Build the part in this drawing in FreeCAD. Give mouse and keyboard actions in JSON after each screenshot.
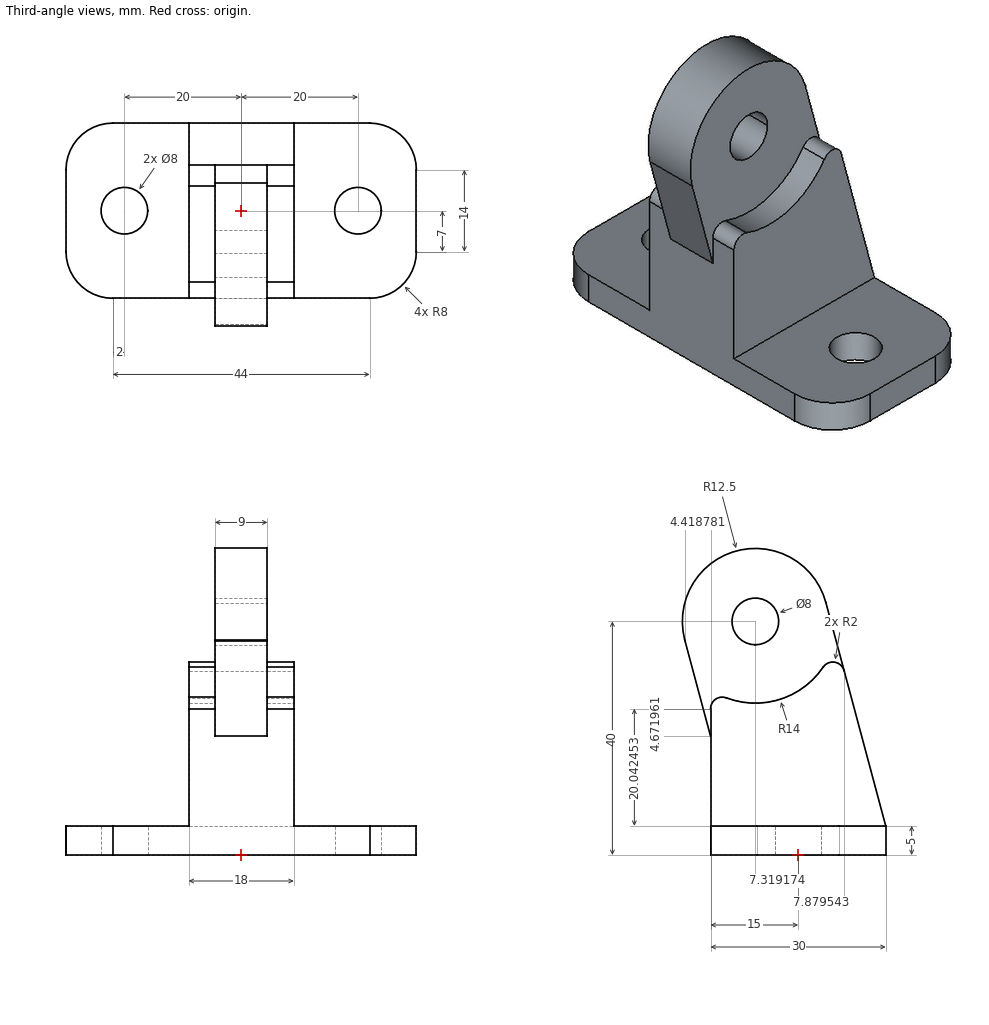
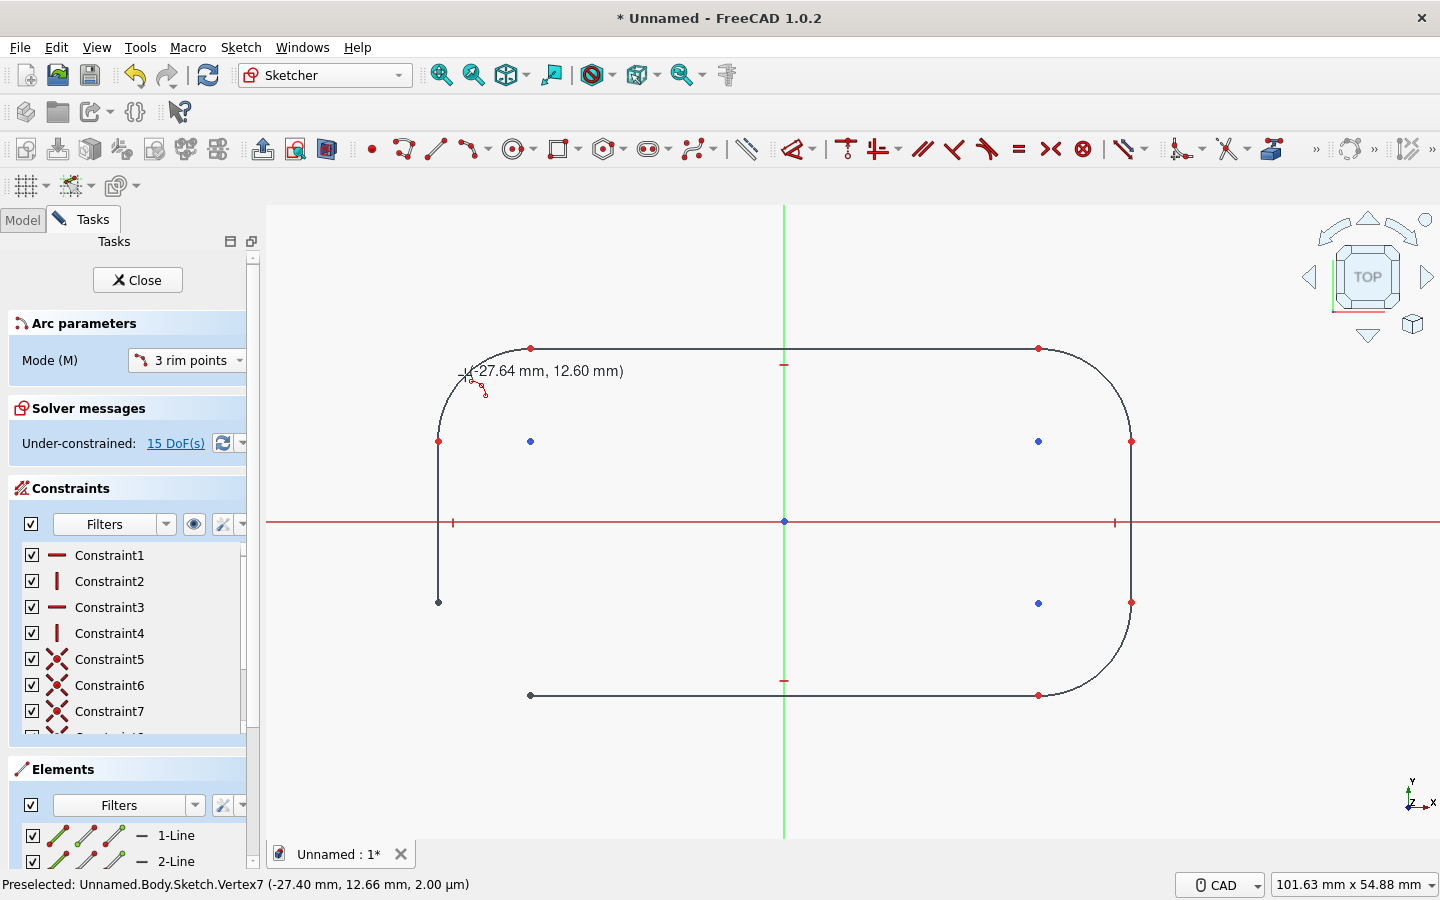
{"action": "left_click", "coordinate": [438, 603]}
{"action": "left_click", "coordinate": [530, 696]}
{"action": "left_click", "coordinate": [465, 668]}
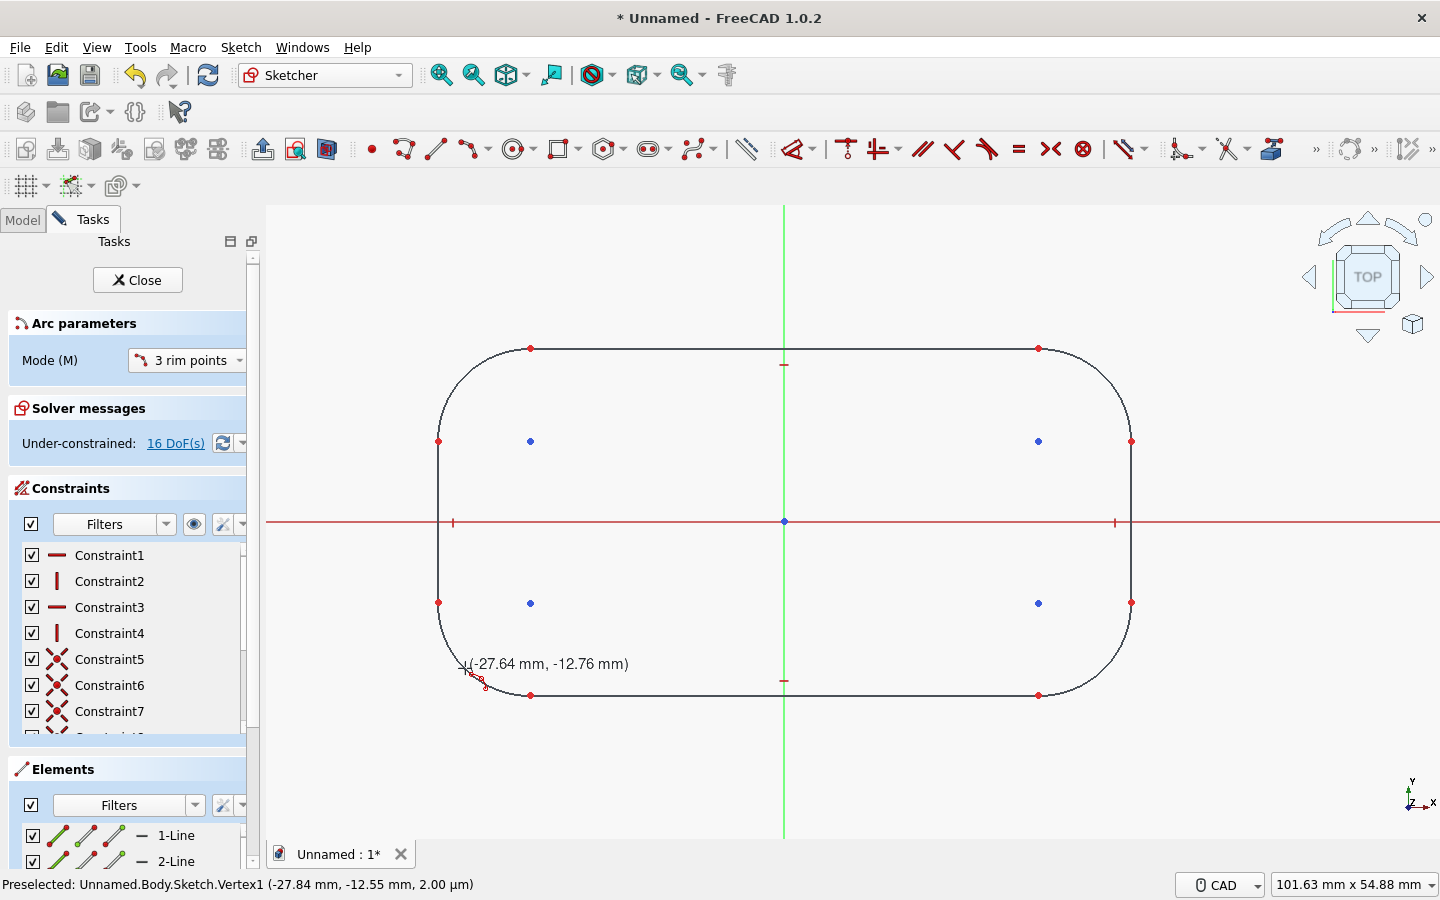
{"action": "left_click", "coordinate": [514, 150]}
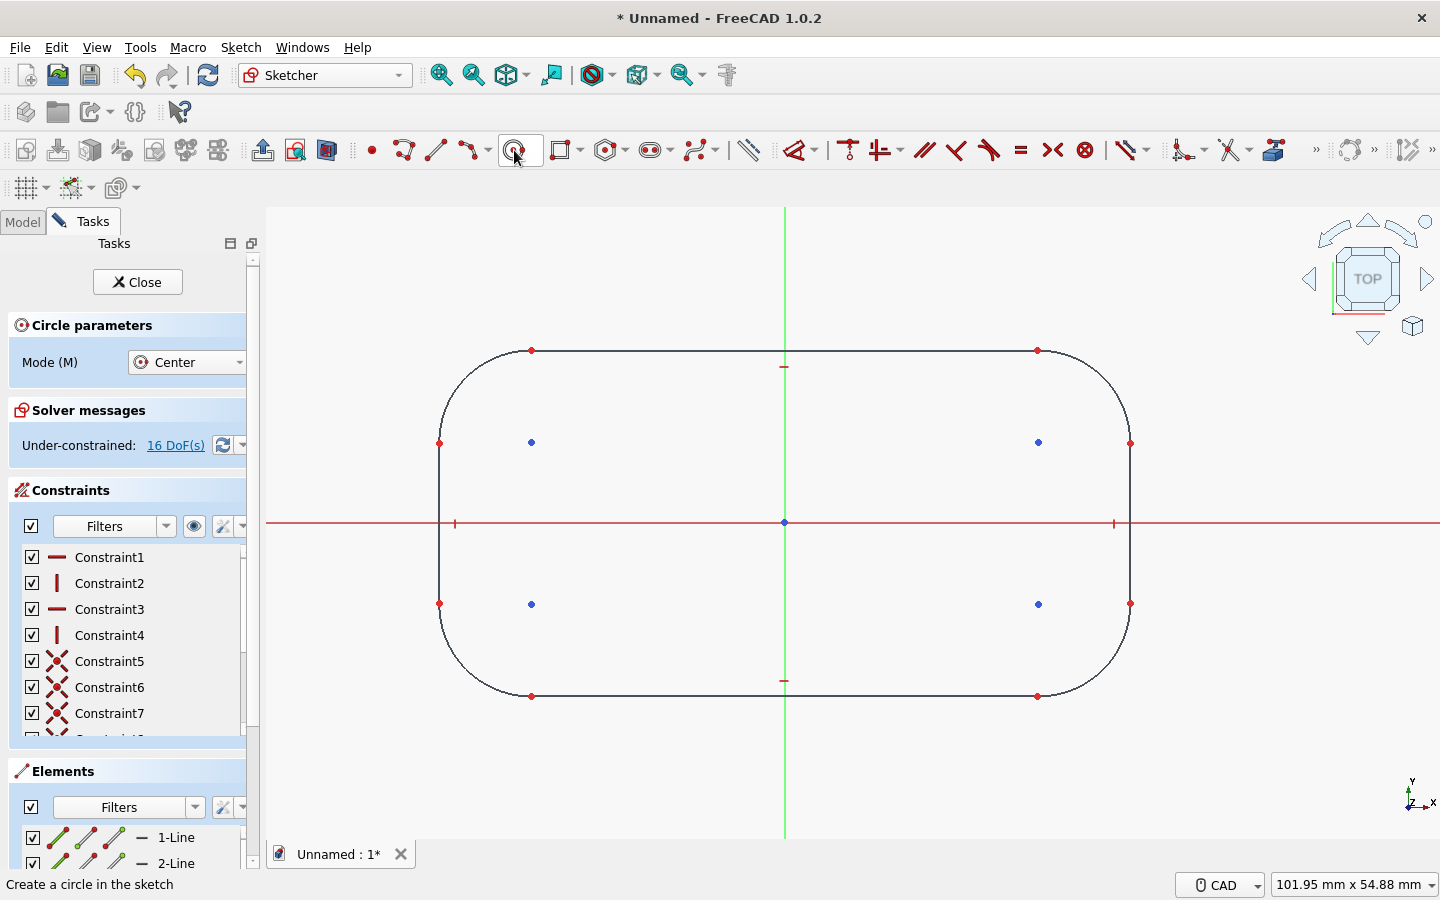
{"action": "left_click", "coordinate": [554, 523]}
{"action": "left_click", "coordinate": [587, 490]}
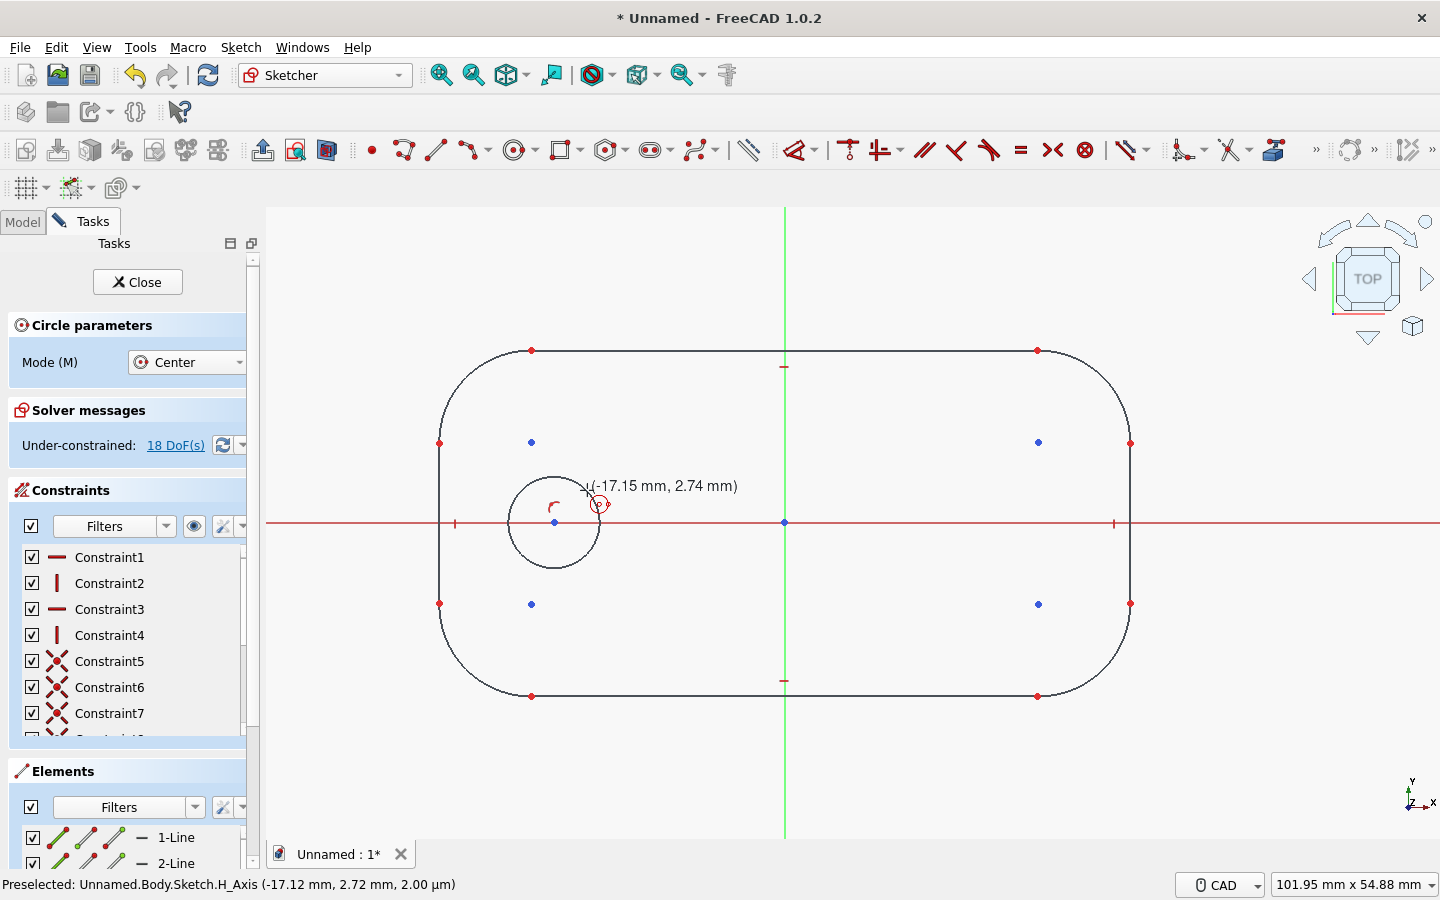
{"action": "left_click", "coordinate": [1015, 523]}
{"action": "left_click", "coordinate": [1047, 490]}
{"action": "key", "text": "Escape"}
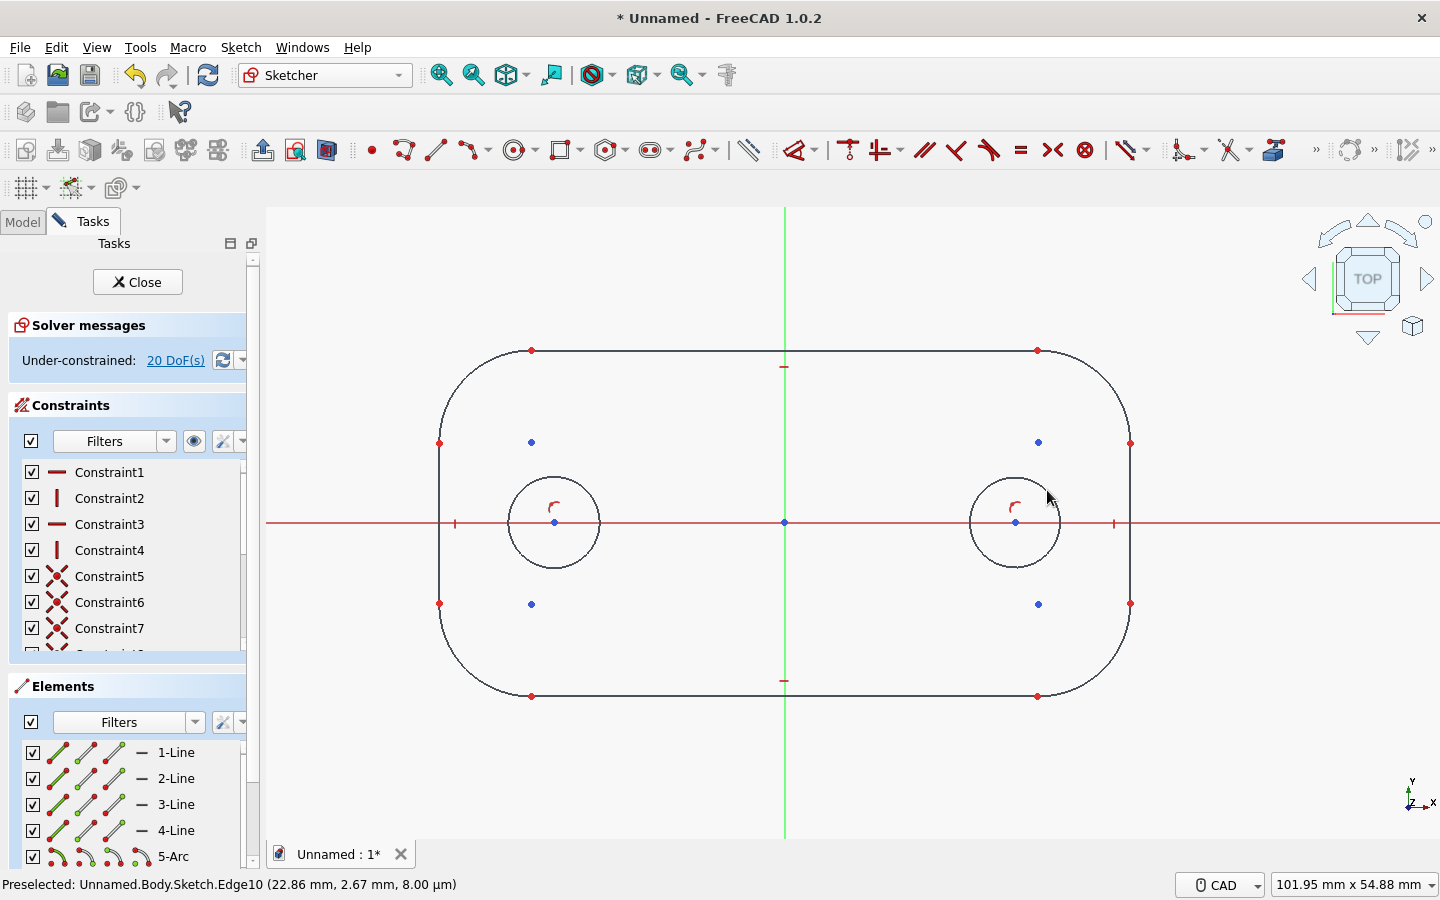
{"action": "left_click", "coordinate": [683, 696]}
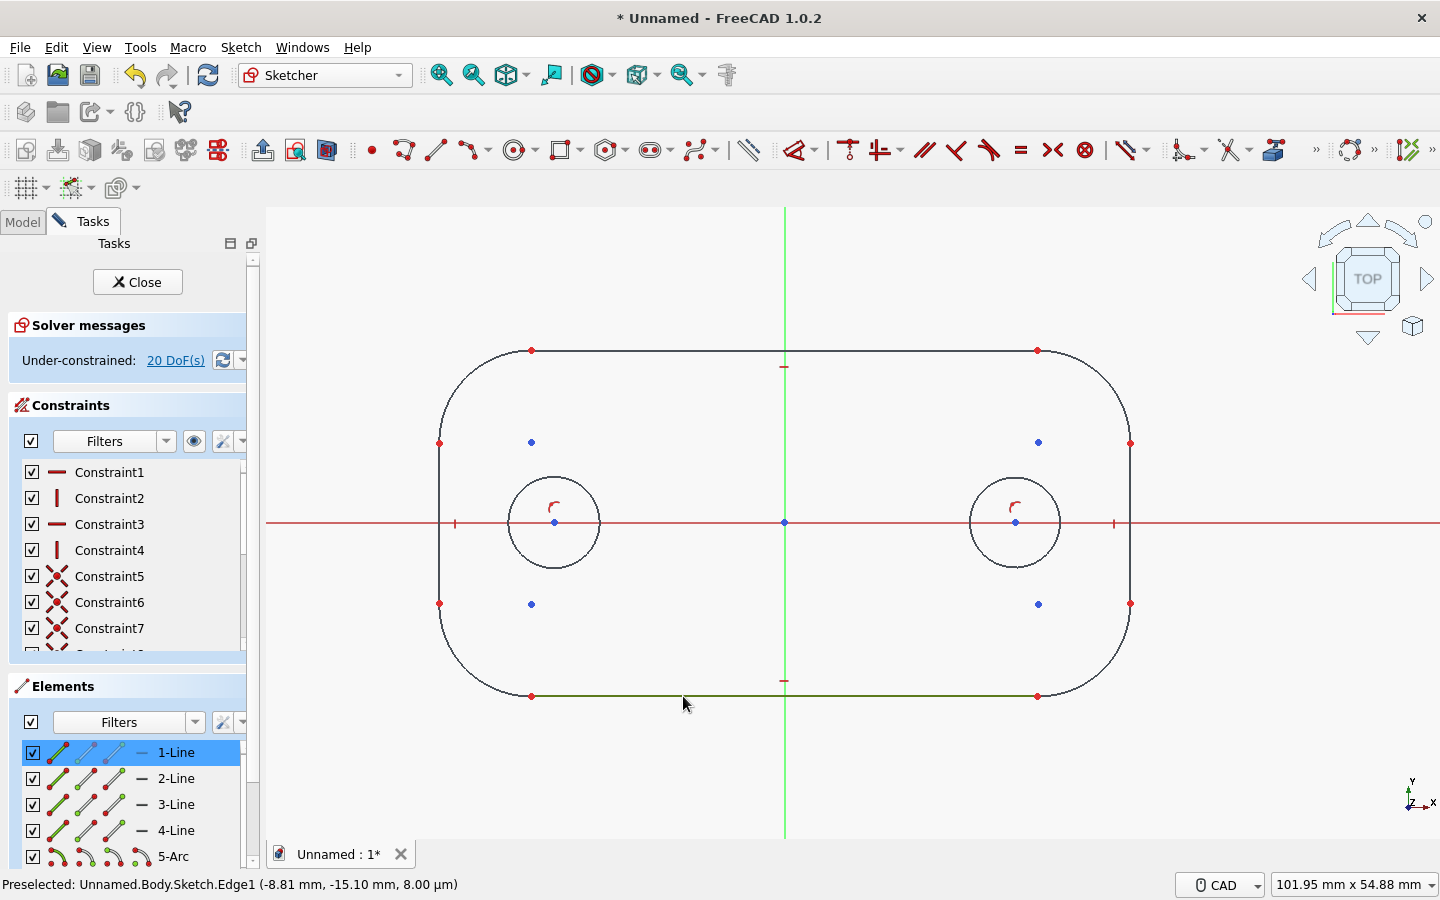
{"action": "left_click", "coordinate": [1080, 687]}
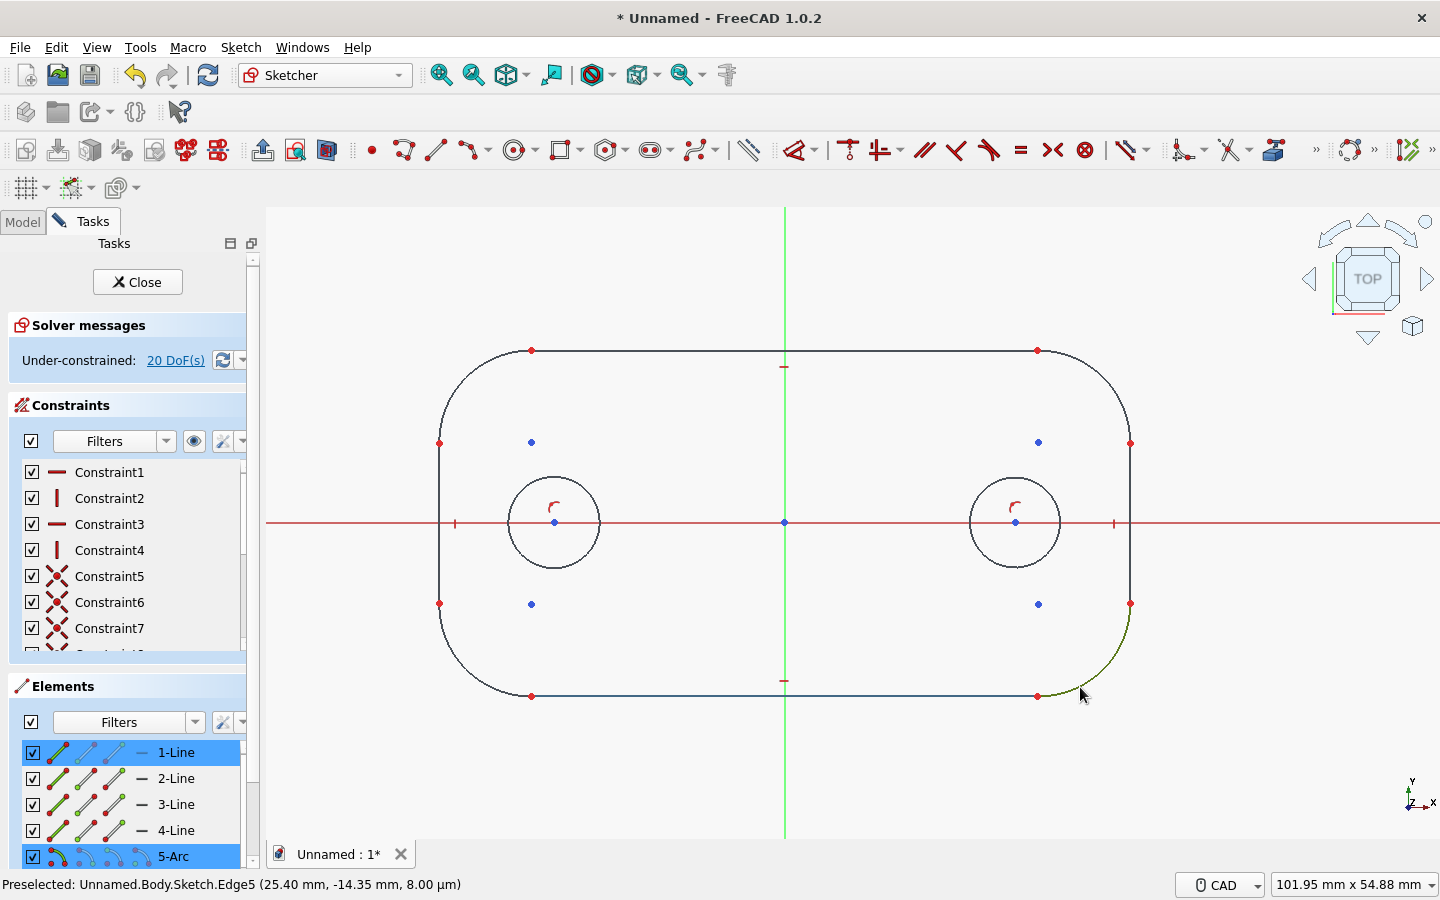
{"action": "left_click", "coordinate": [990, 150]}